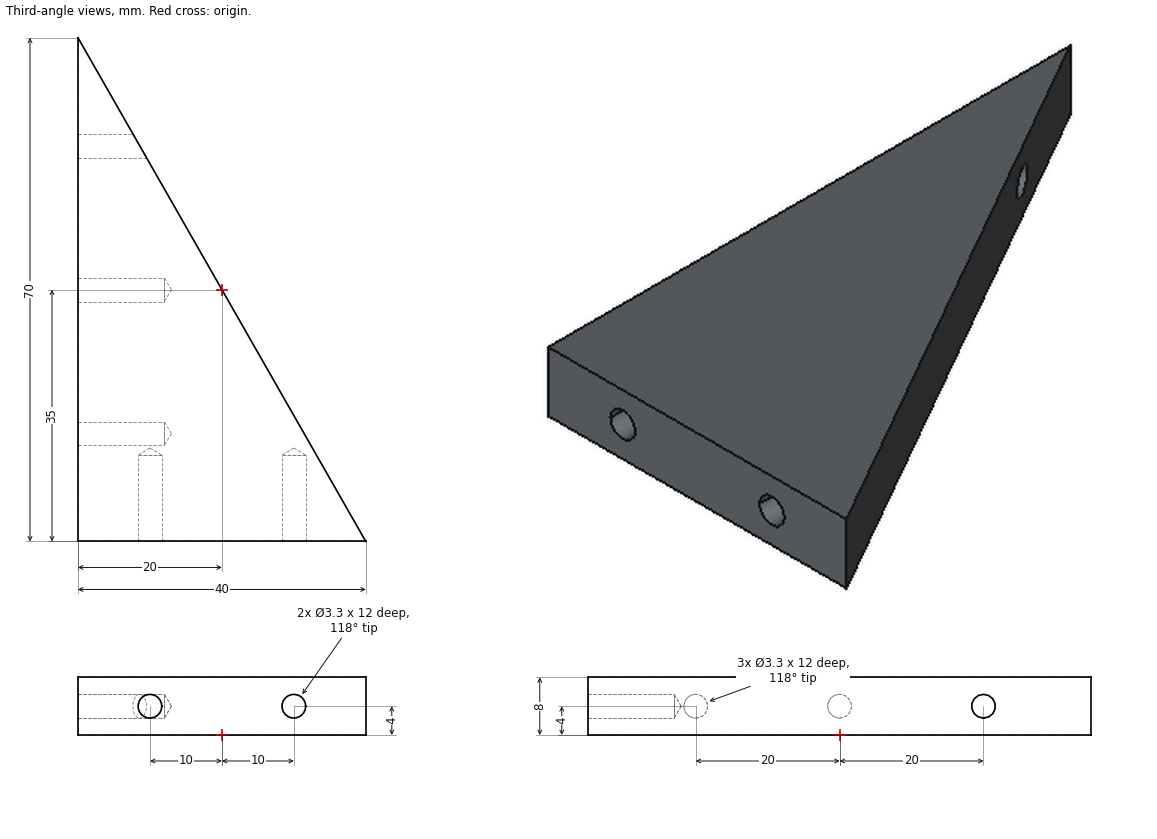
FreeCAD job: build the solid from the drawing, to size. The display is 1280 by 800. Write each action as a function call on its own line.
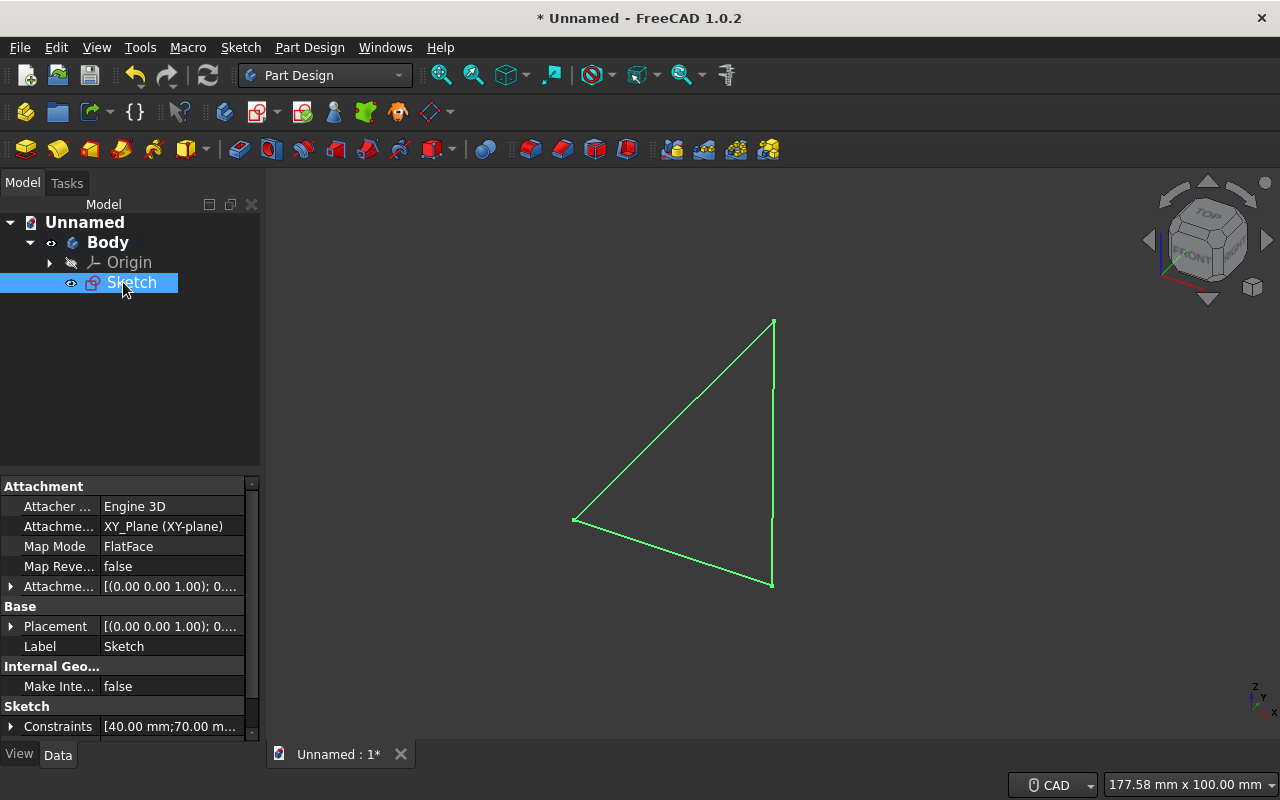
click(26, 150)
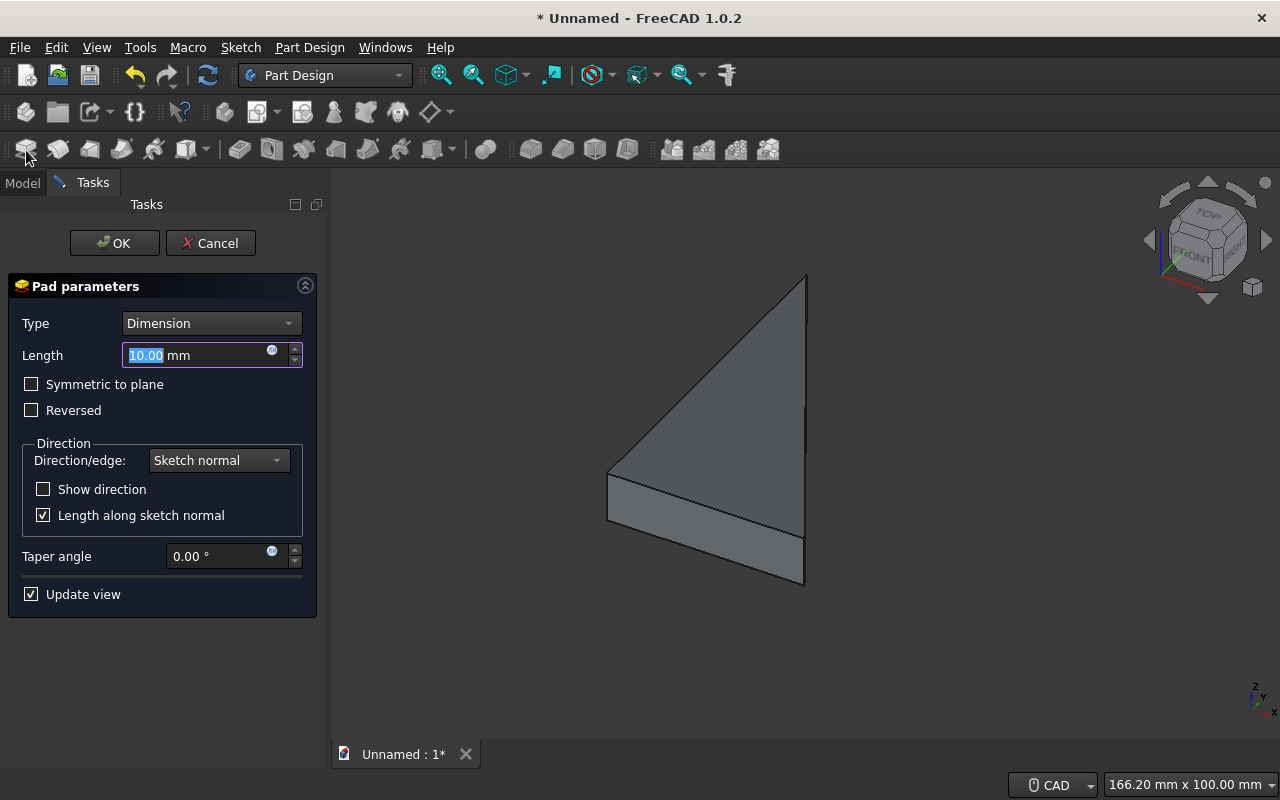
text(8)
key(Tab)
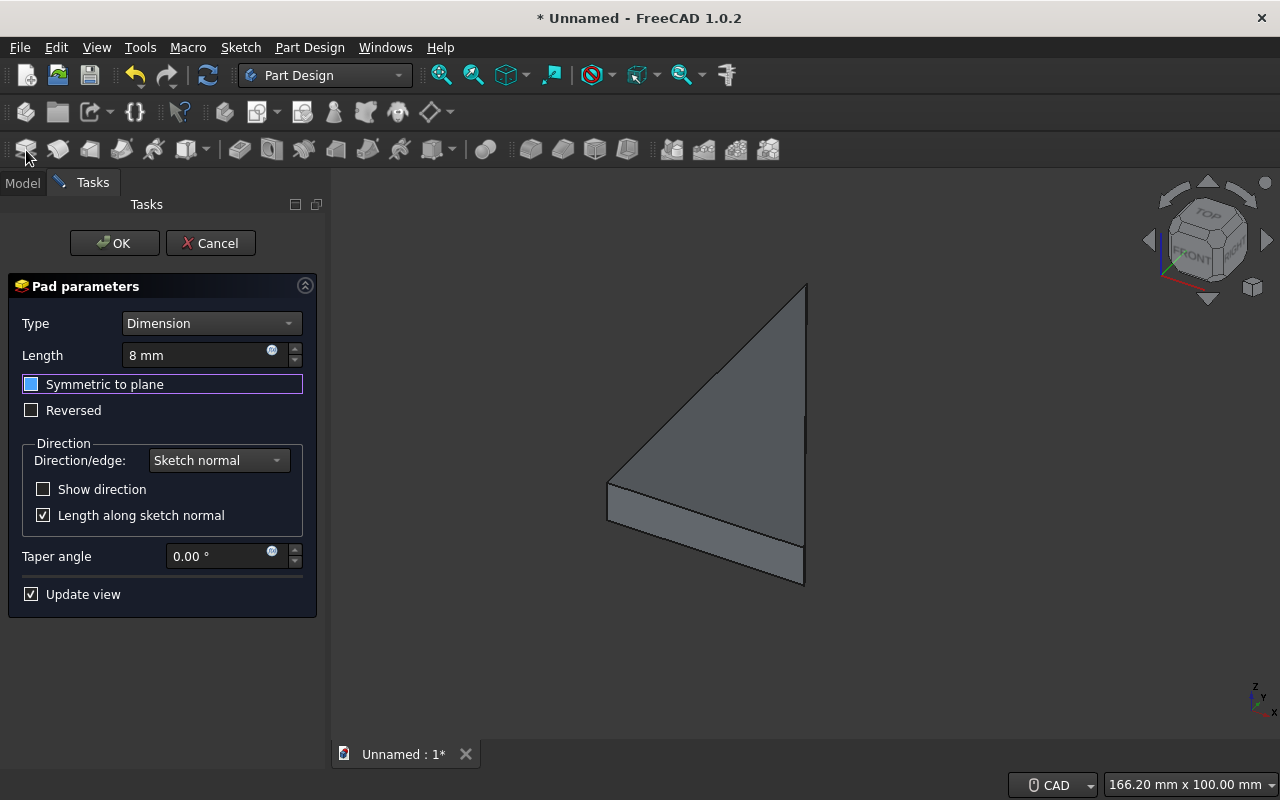
click(115, 243)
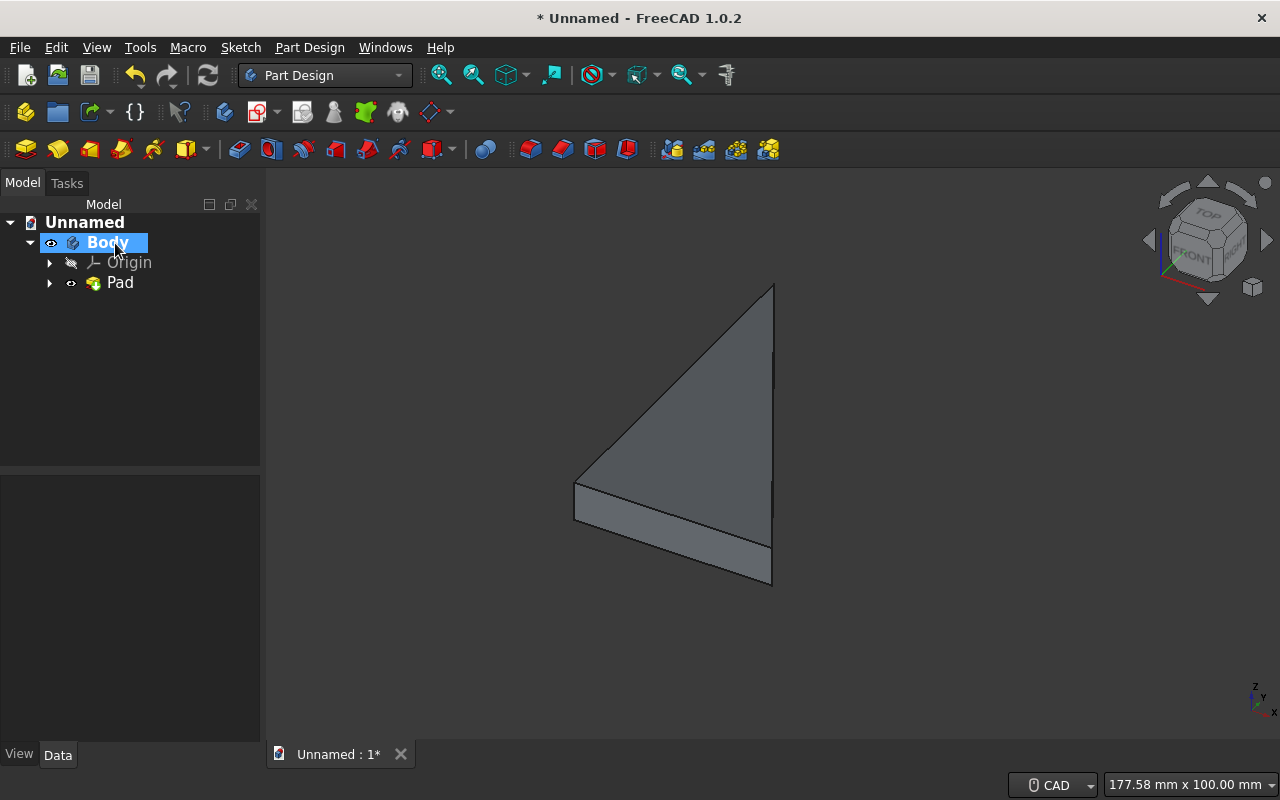
key(6)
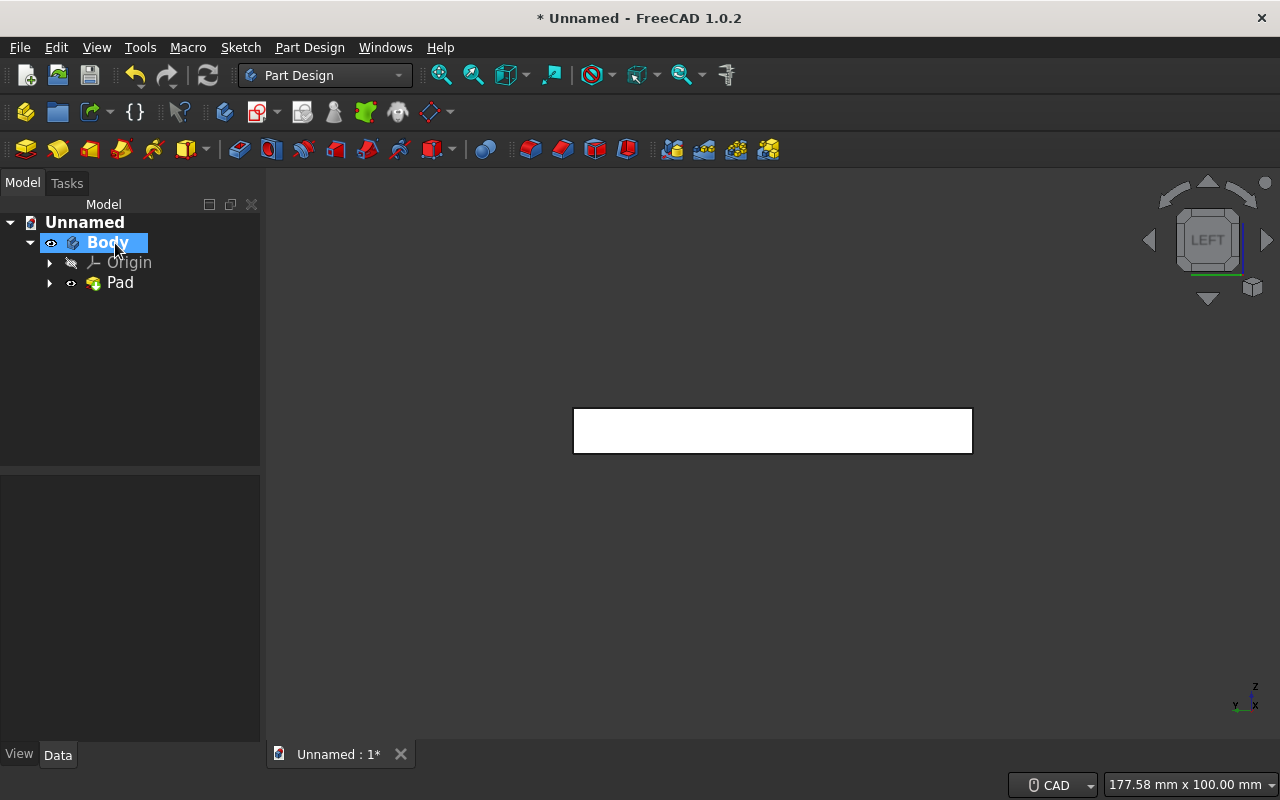
click(442, 76)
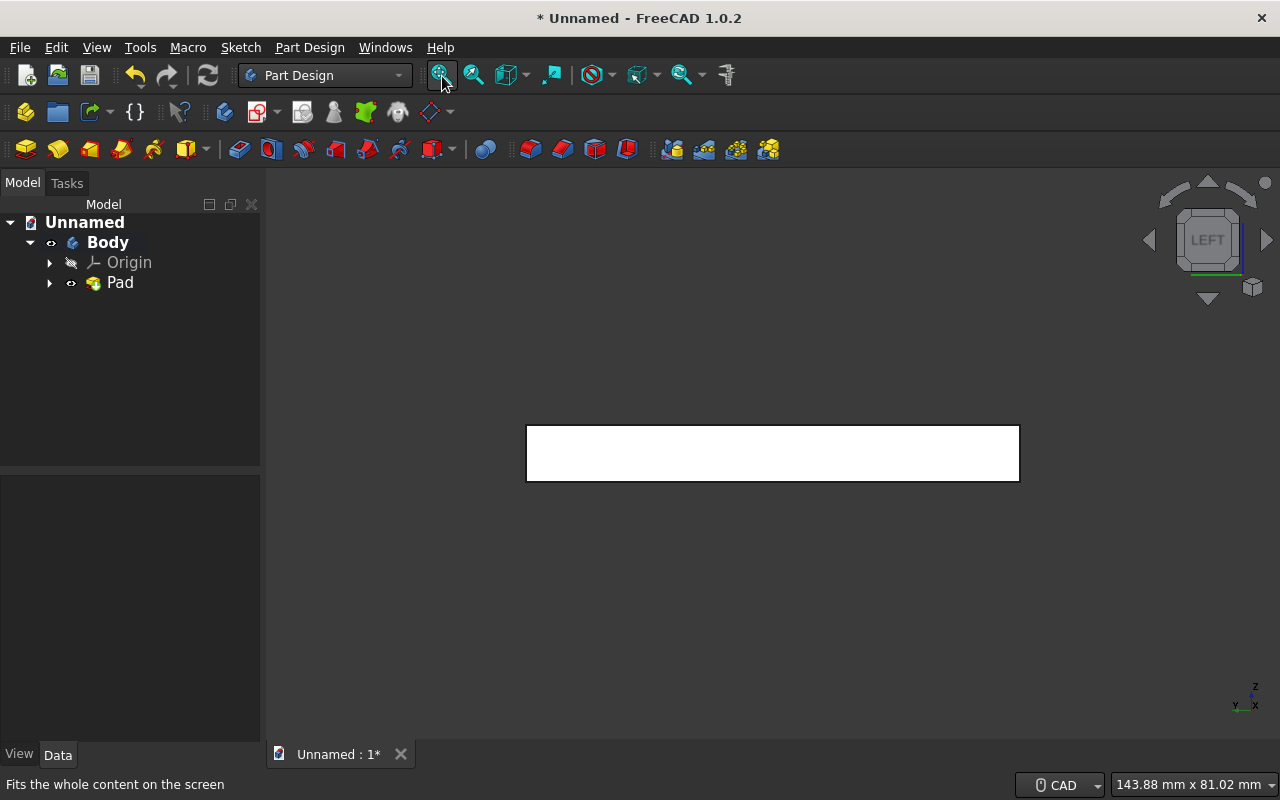
click(562, 452)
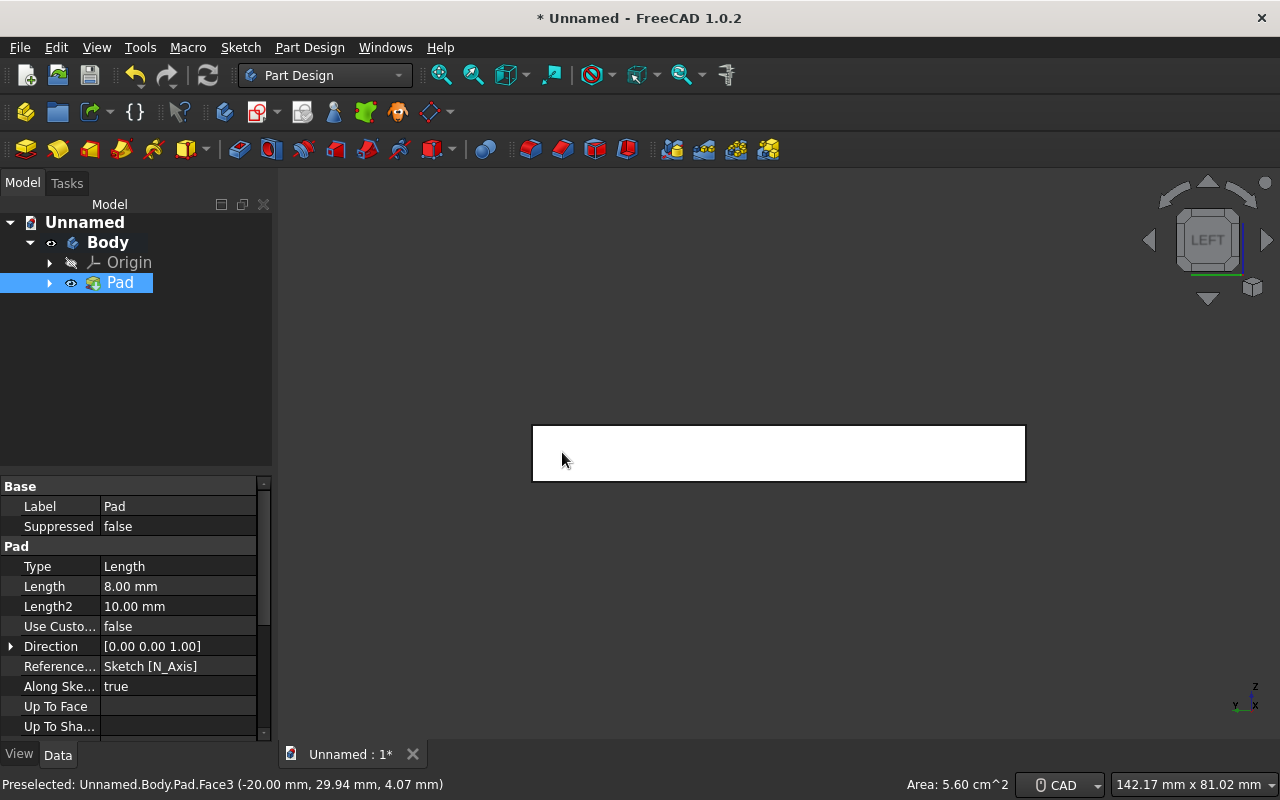
click(258, 112)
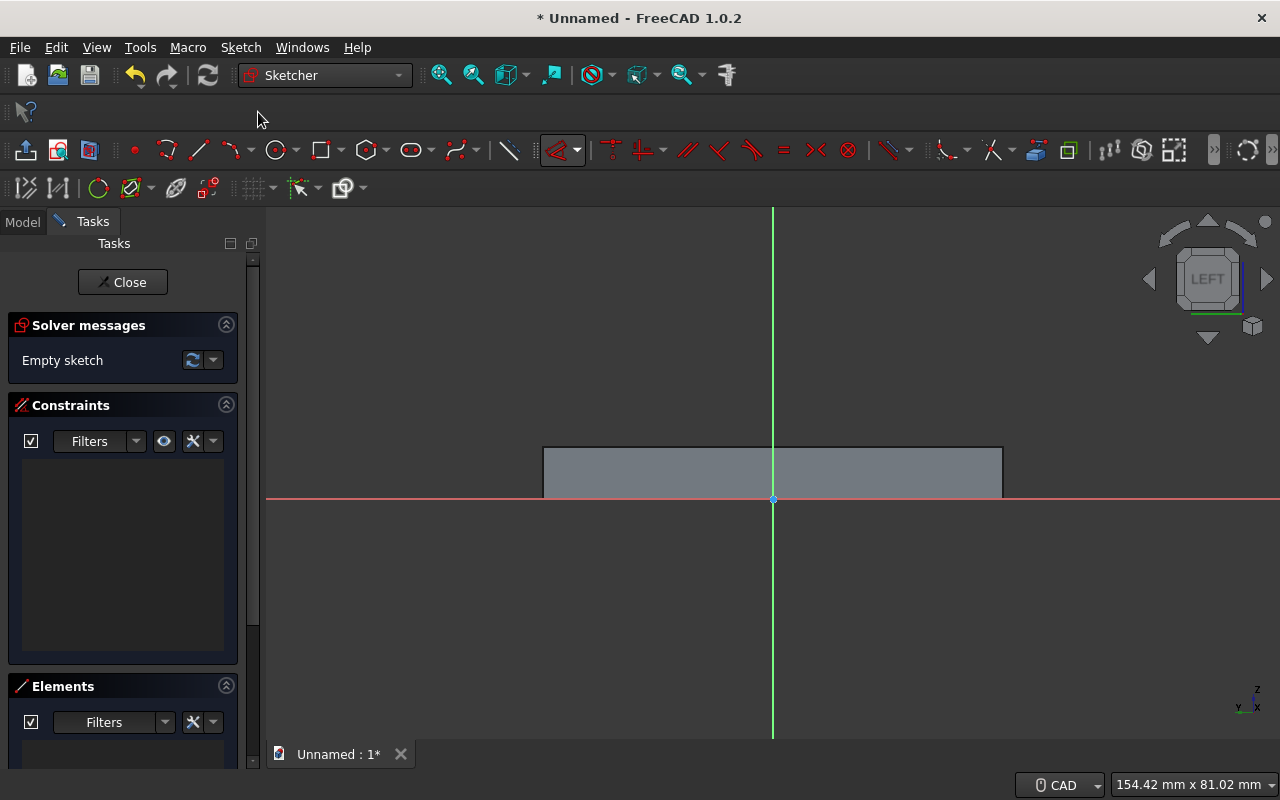
scroll(829, 487, up, 4)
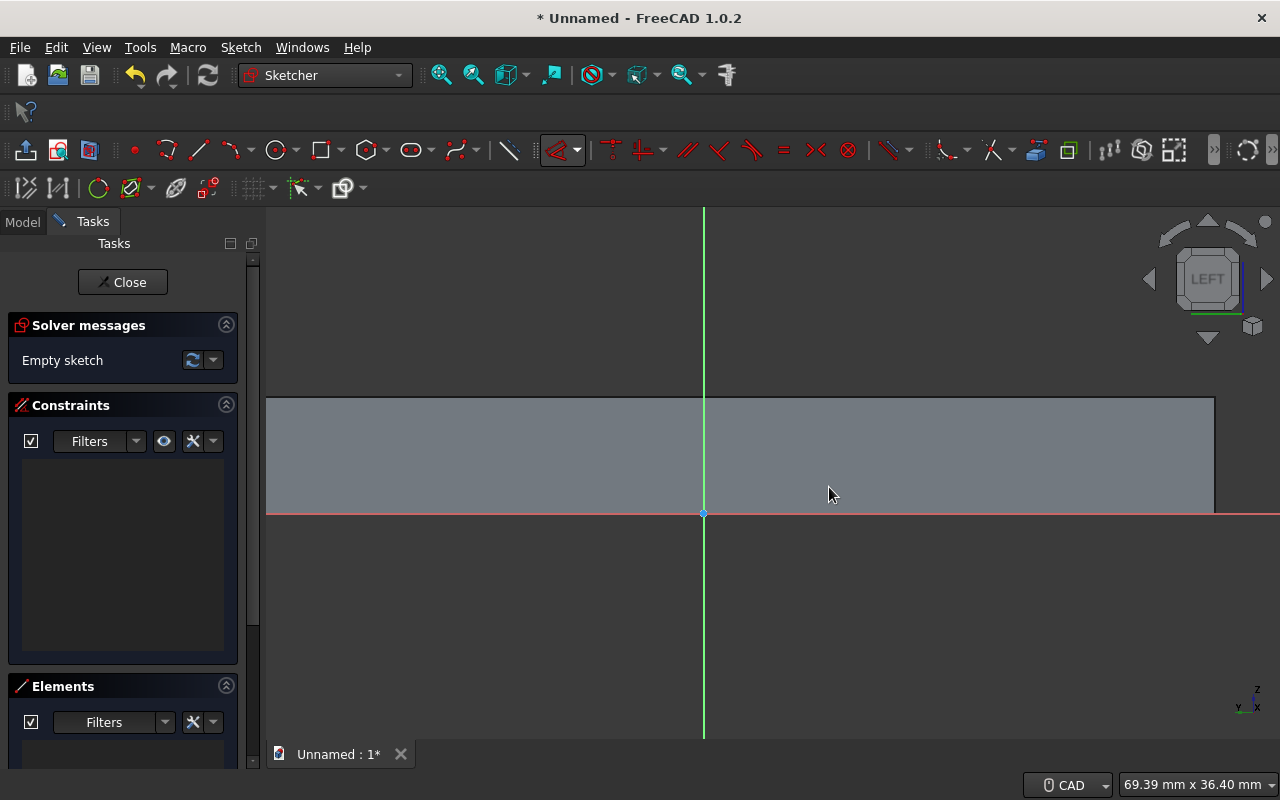
click(276, 150)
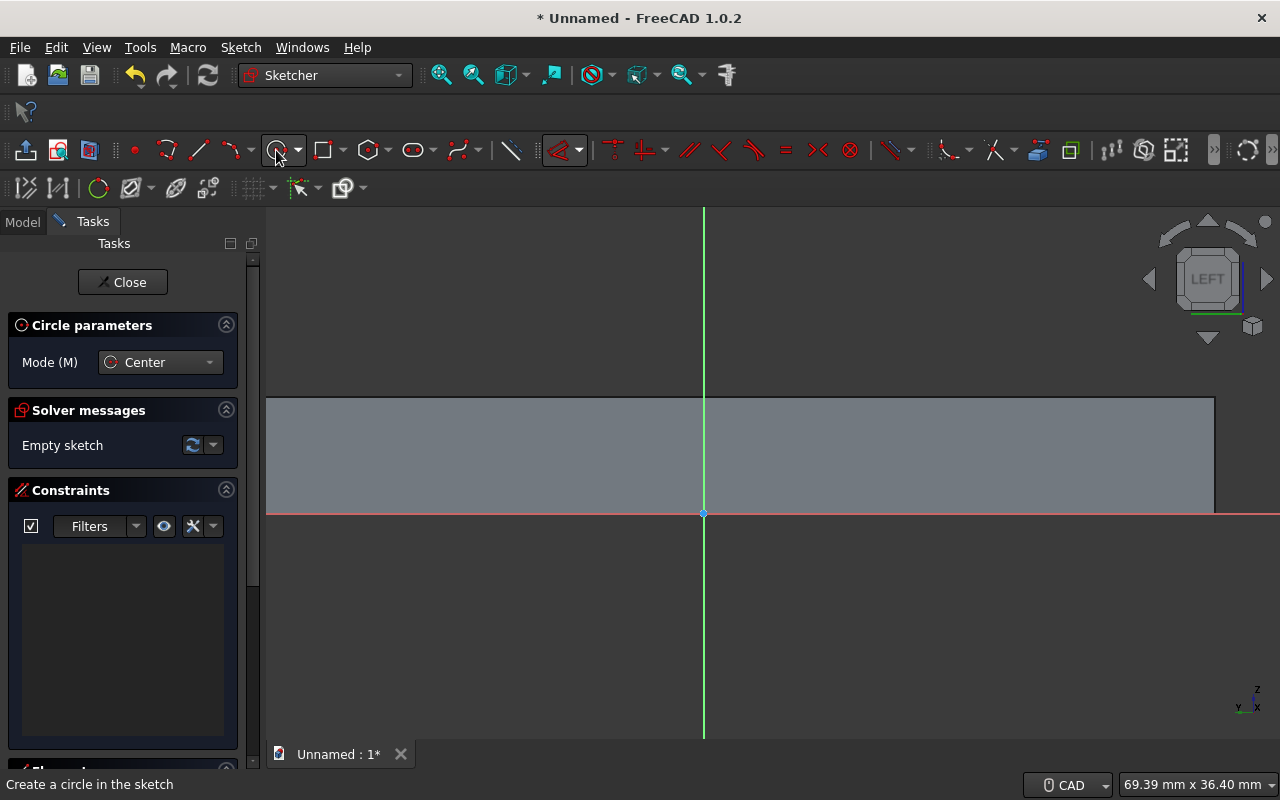
click(996, 455)
click(1013, 438)